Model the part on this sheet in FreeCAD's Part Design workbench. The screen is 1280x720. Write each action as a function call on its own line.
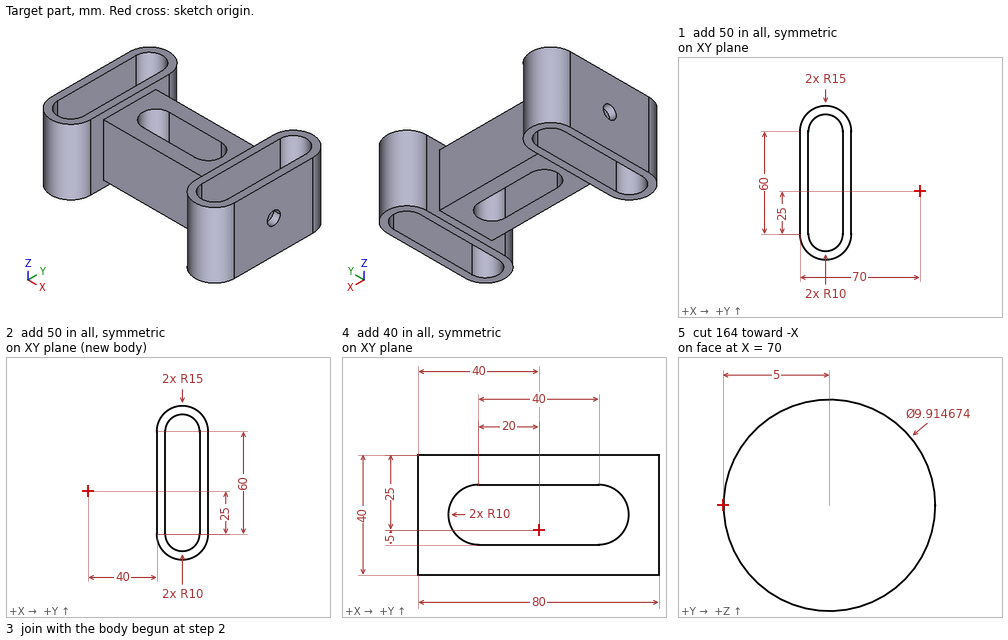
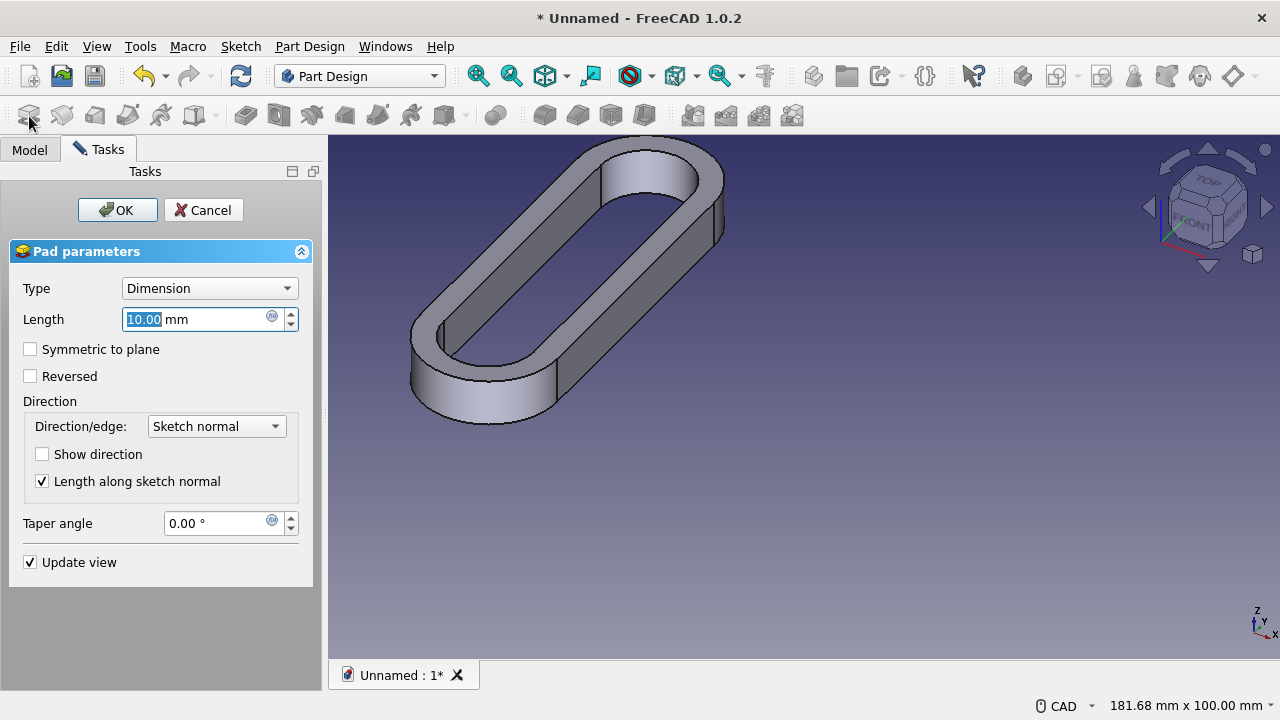
text(50)
key(Tab)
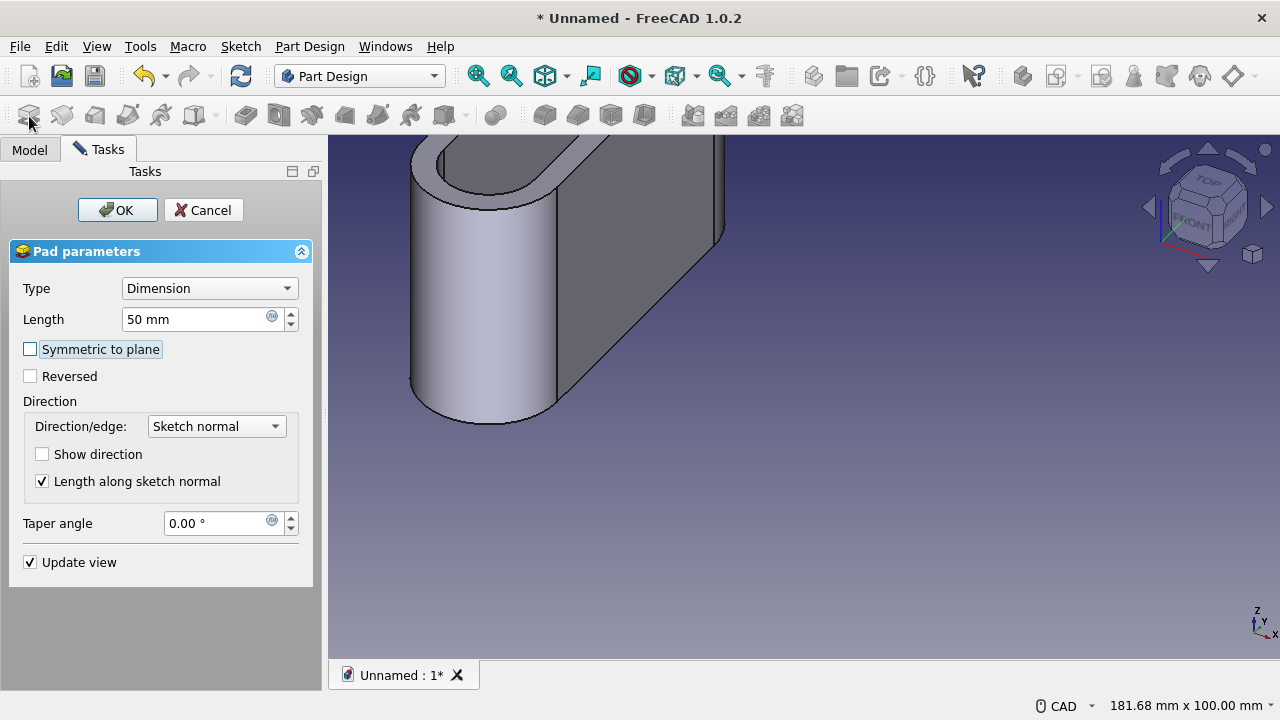
click(31, 349)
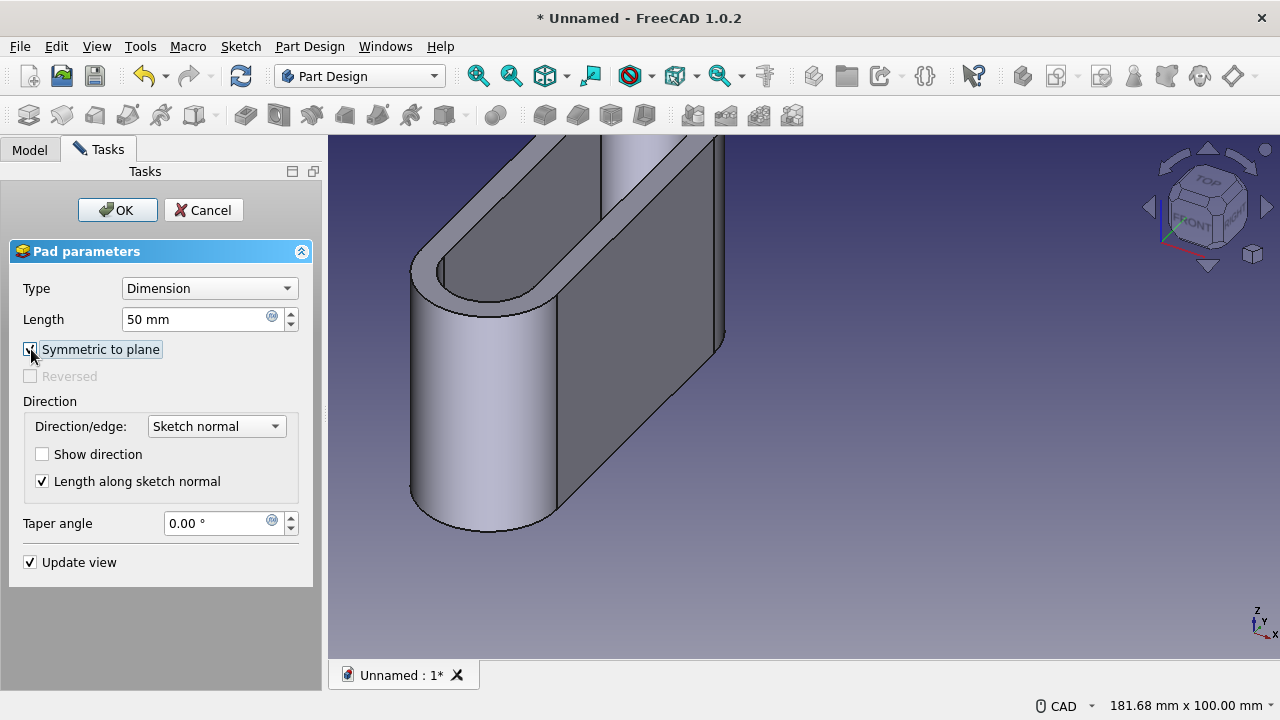
click(118, 210)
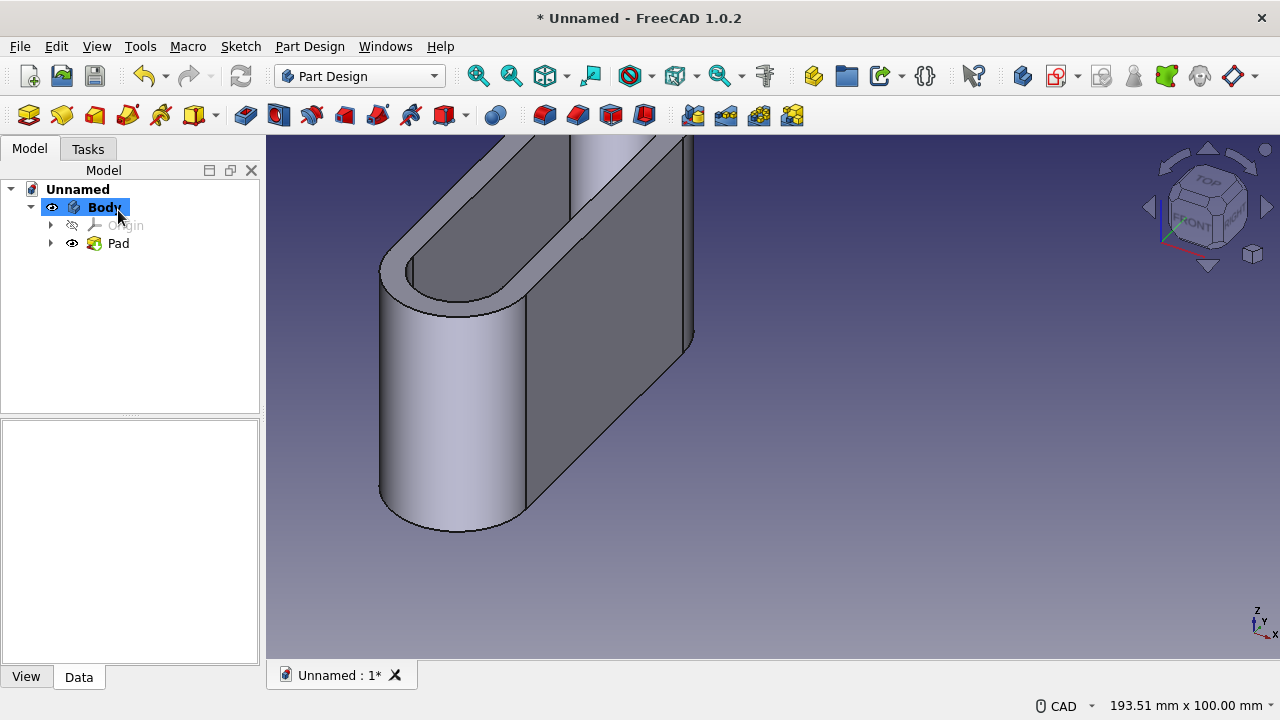
click(479, 76)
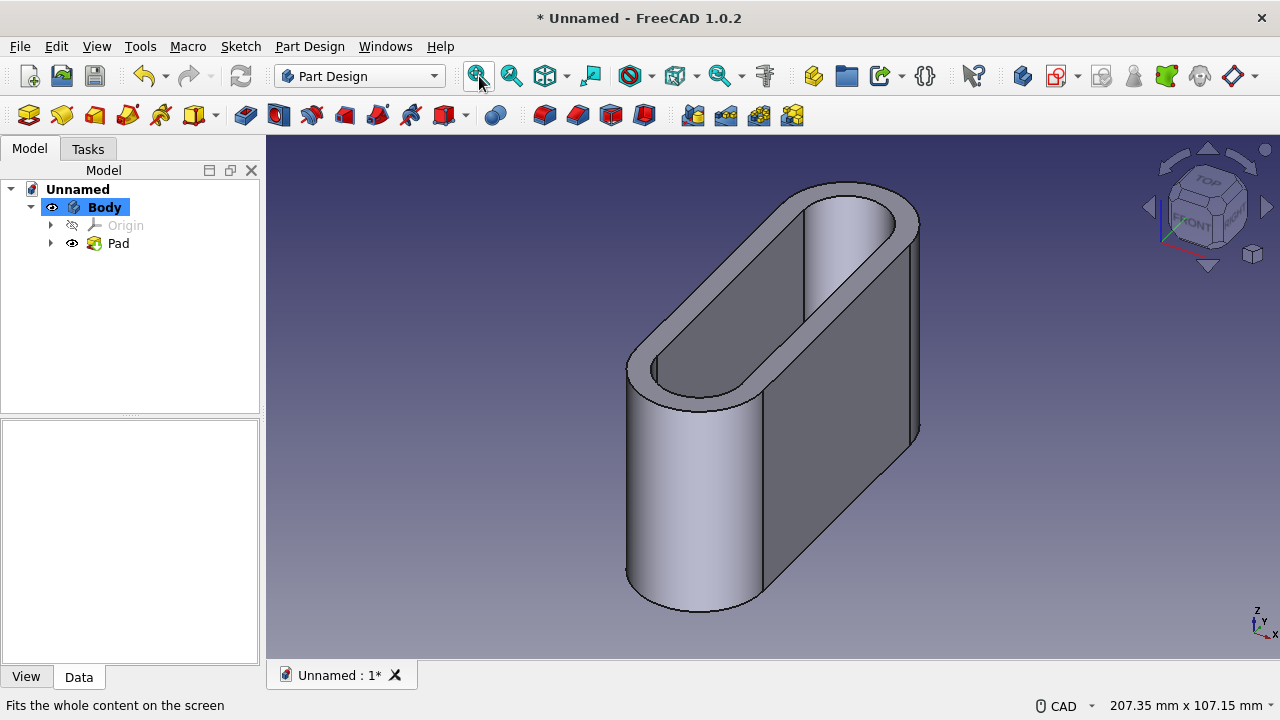
click(1023, 76)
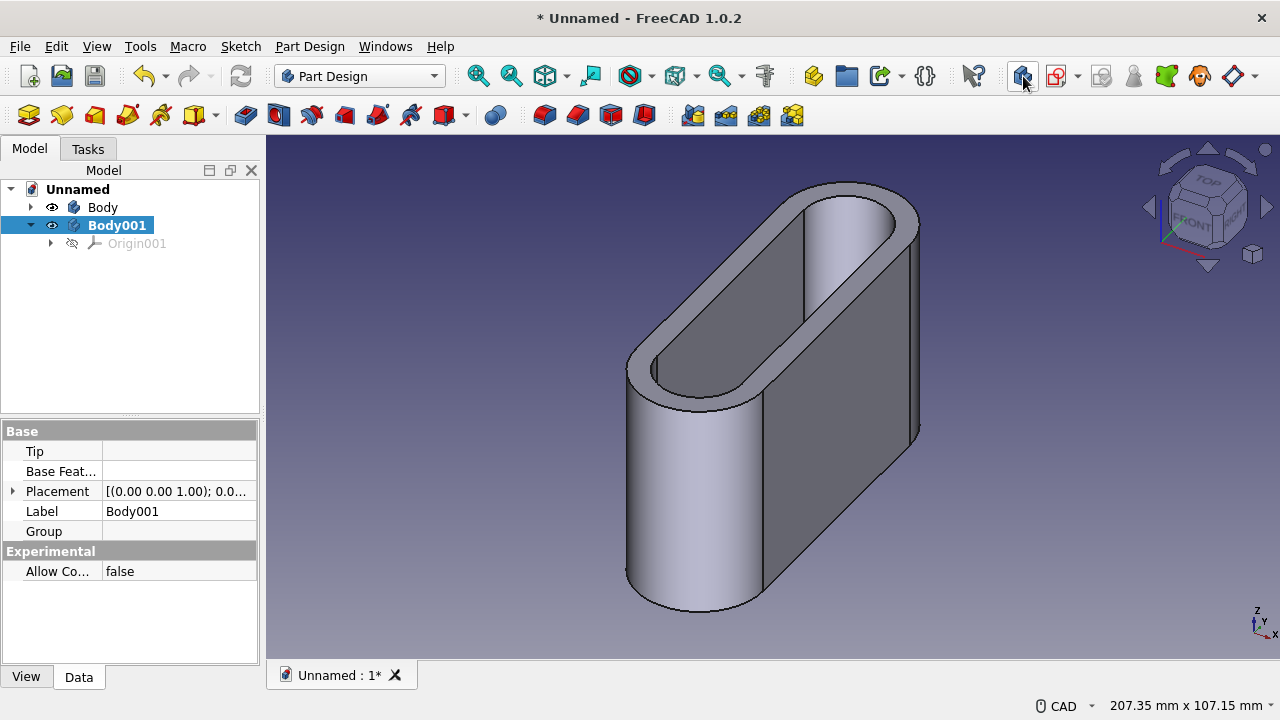
click(306, 619)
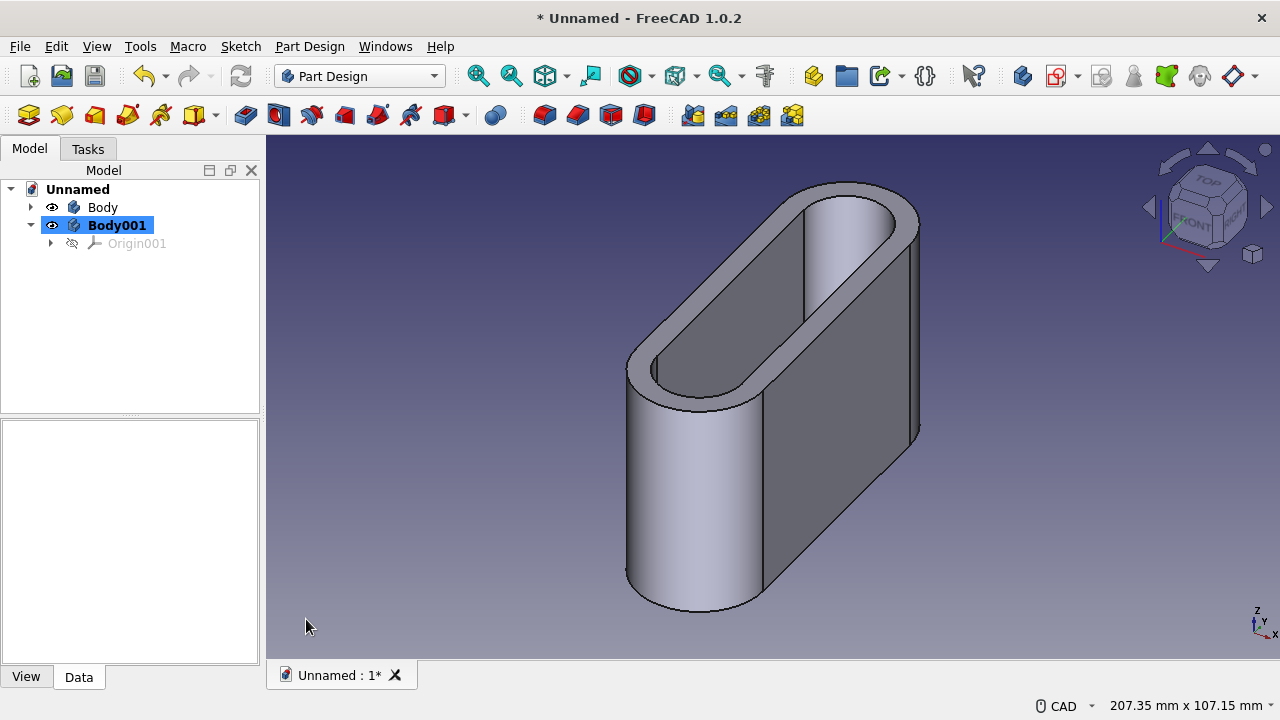
click(1056, 76)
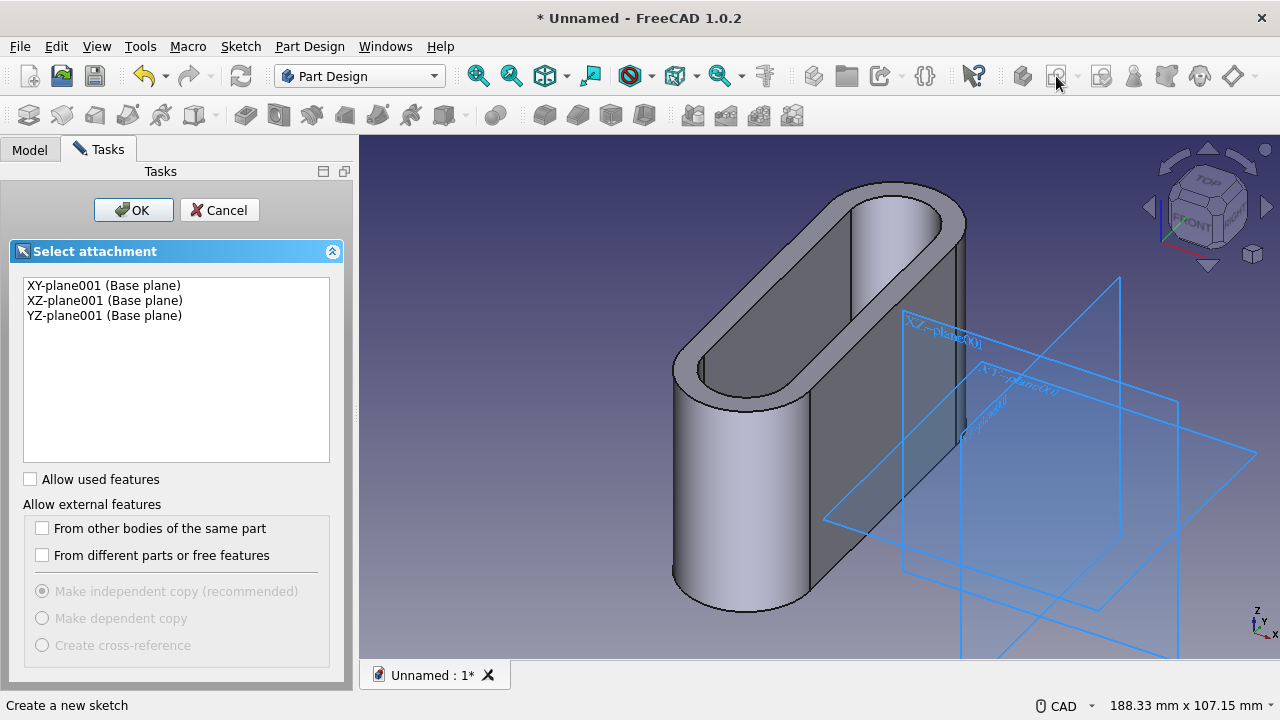
click(84, 286)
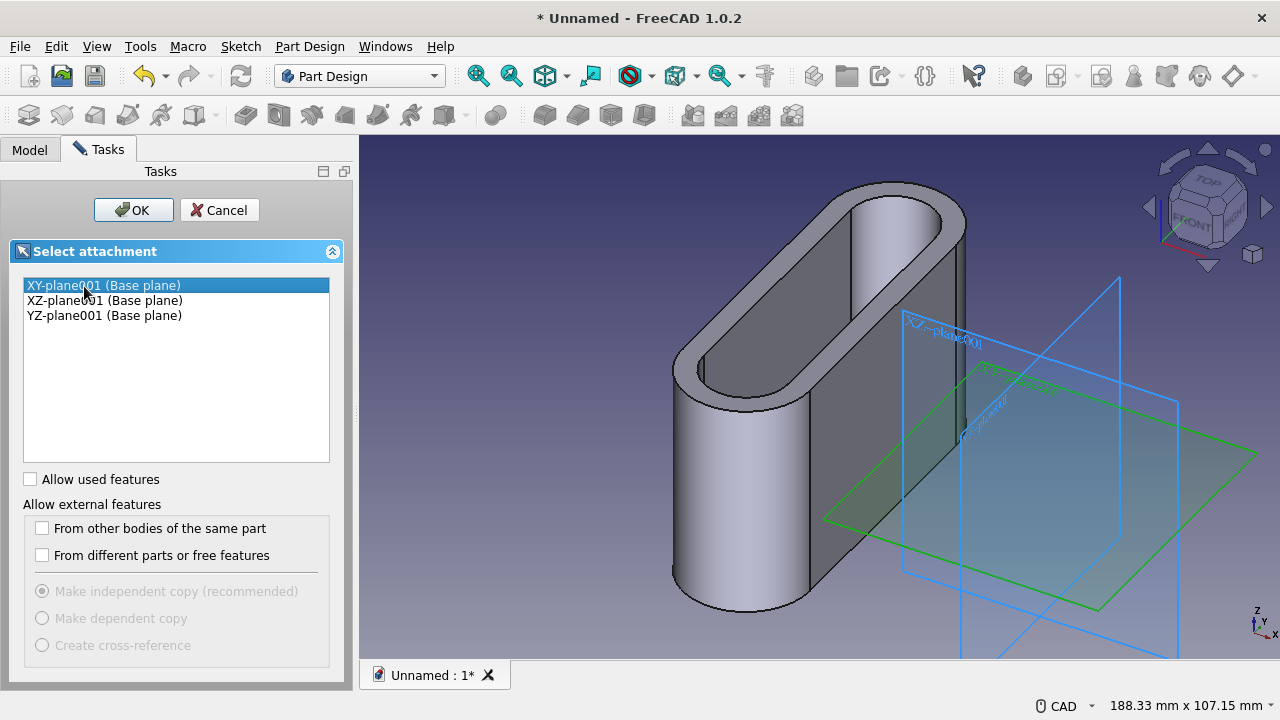
click(134, 210)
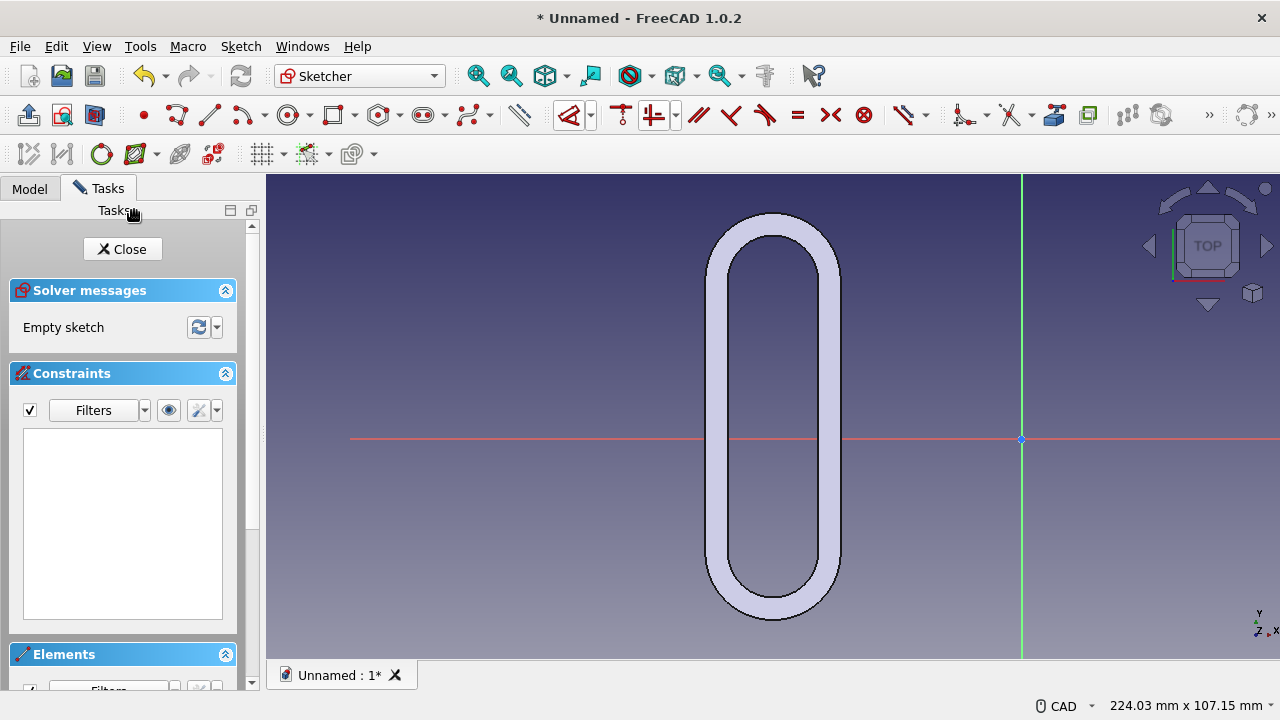
scroll(294, 416, down, 2)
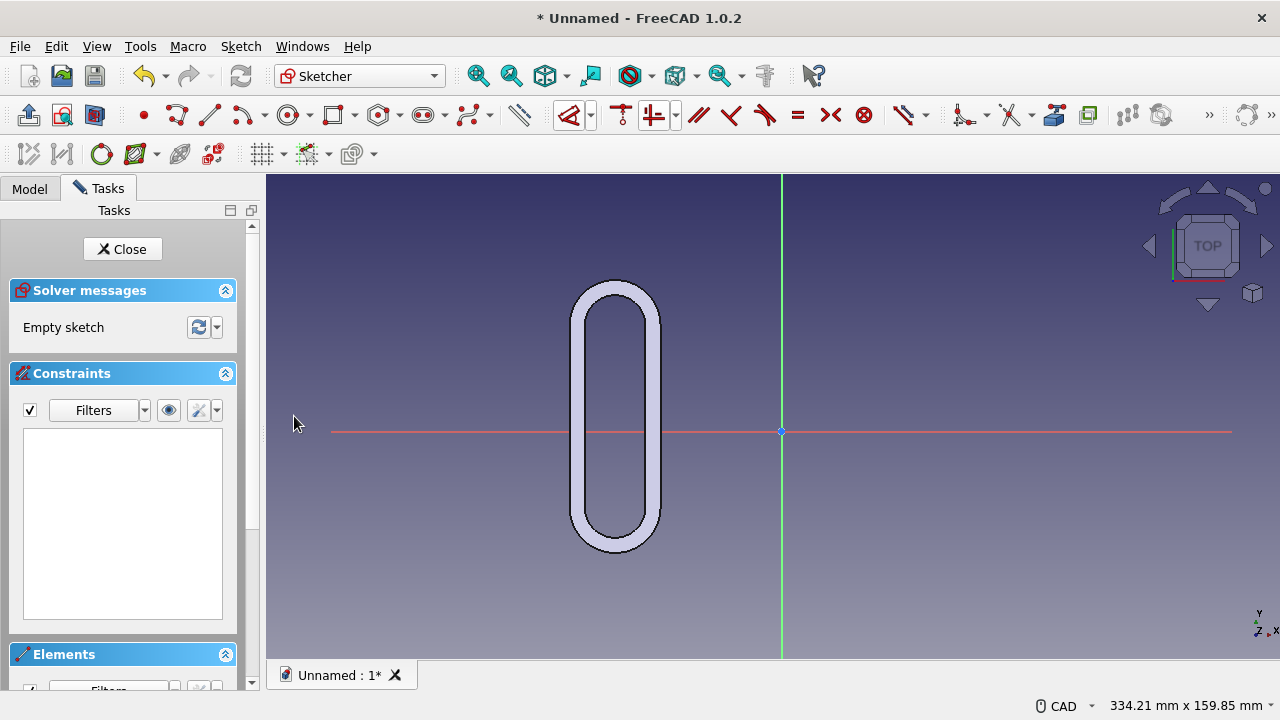
click(422, 116)